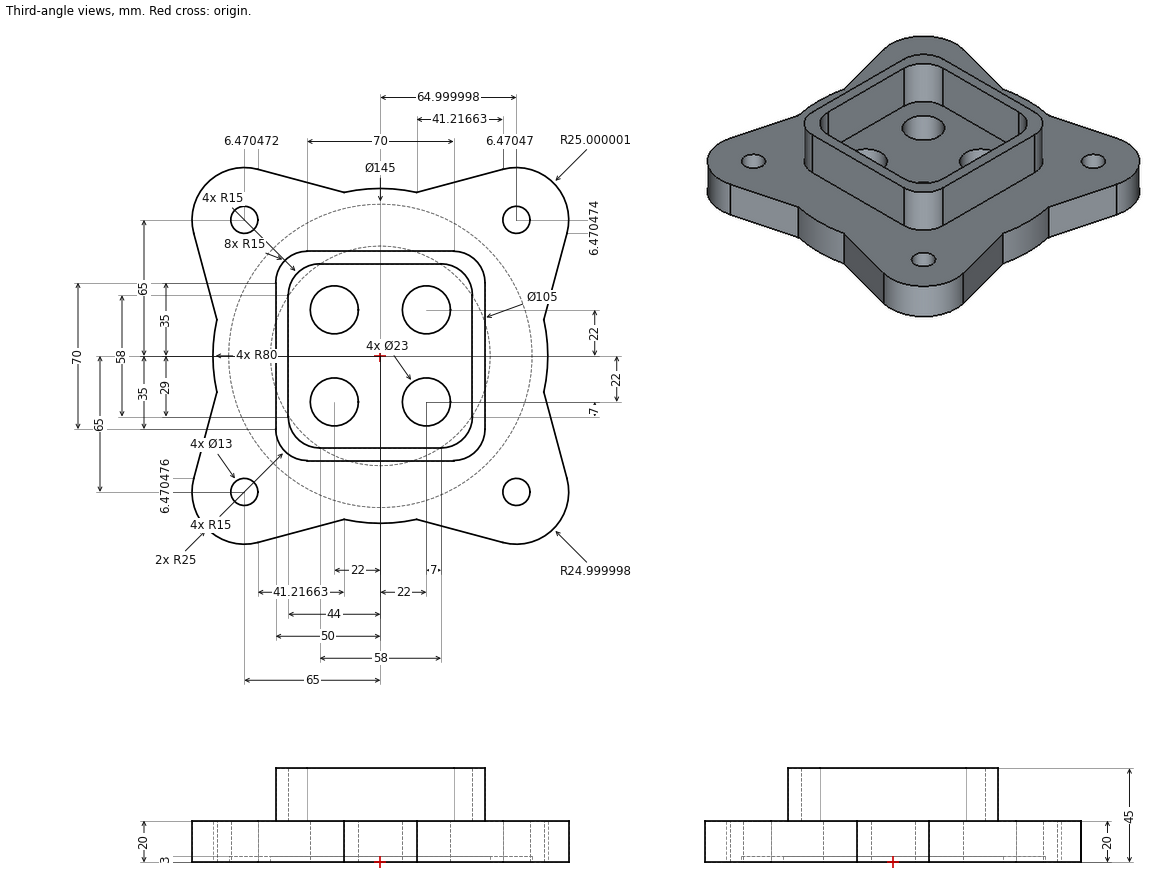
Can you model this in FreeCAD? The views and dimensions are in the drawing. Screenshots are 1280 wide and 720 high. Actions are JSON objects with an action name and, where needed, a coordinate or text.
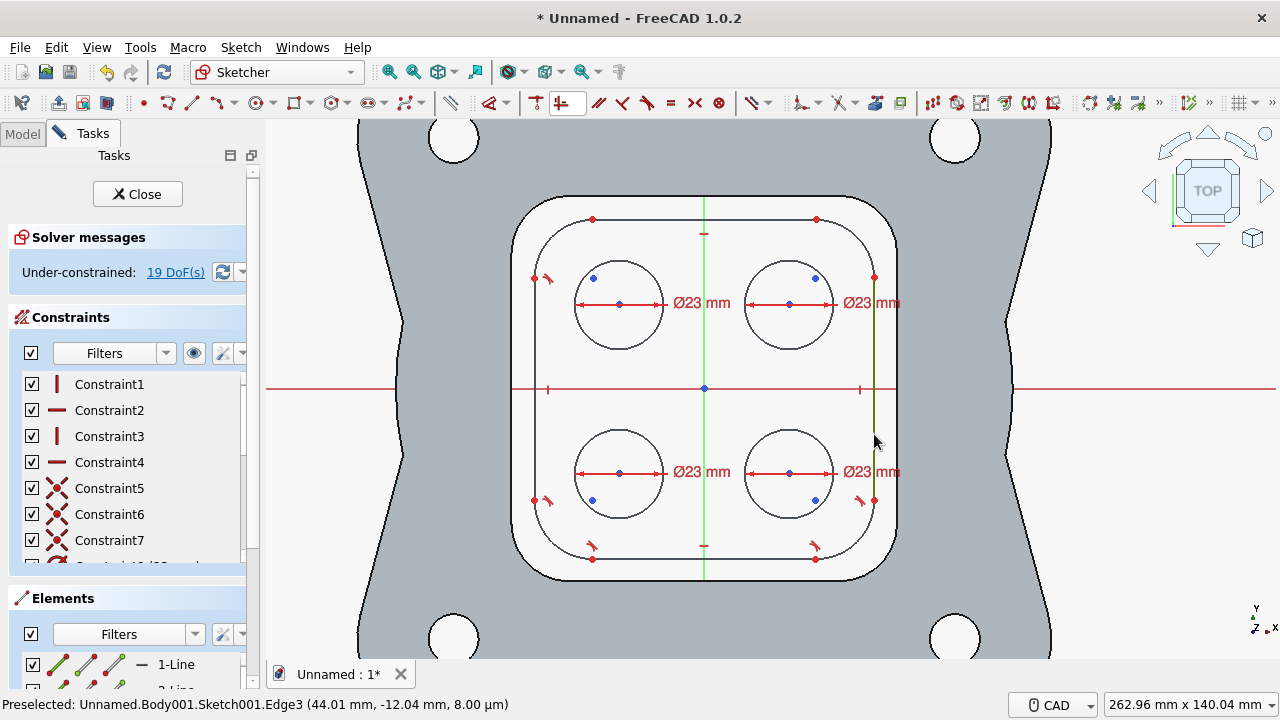
{"action": "left_click", "coordinate": [868, 252]}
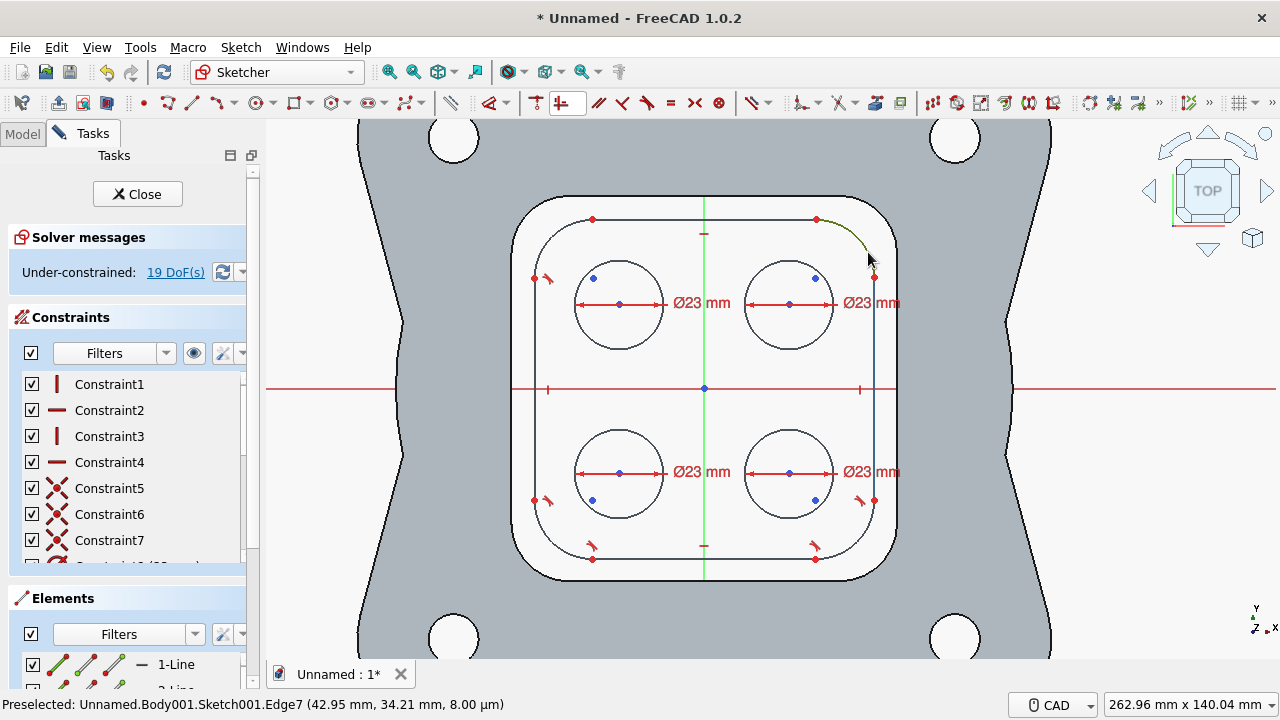
{"action": "key", "text": "t"}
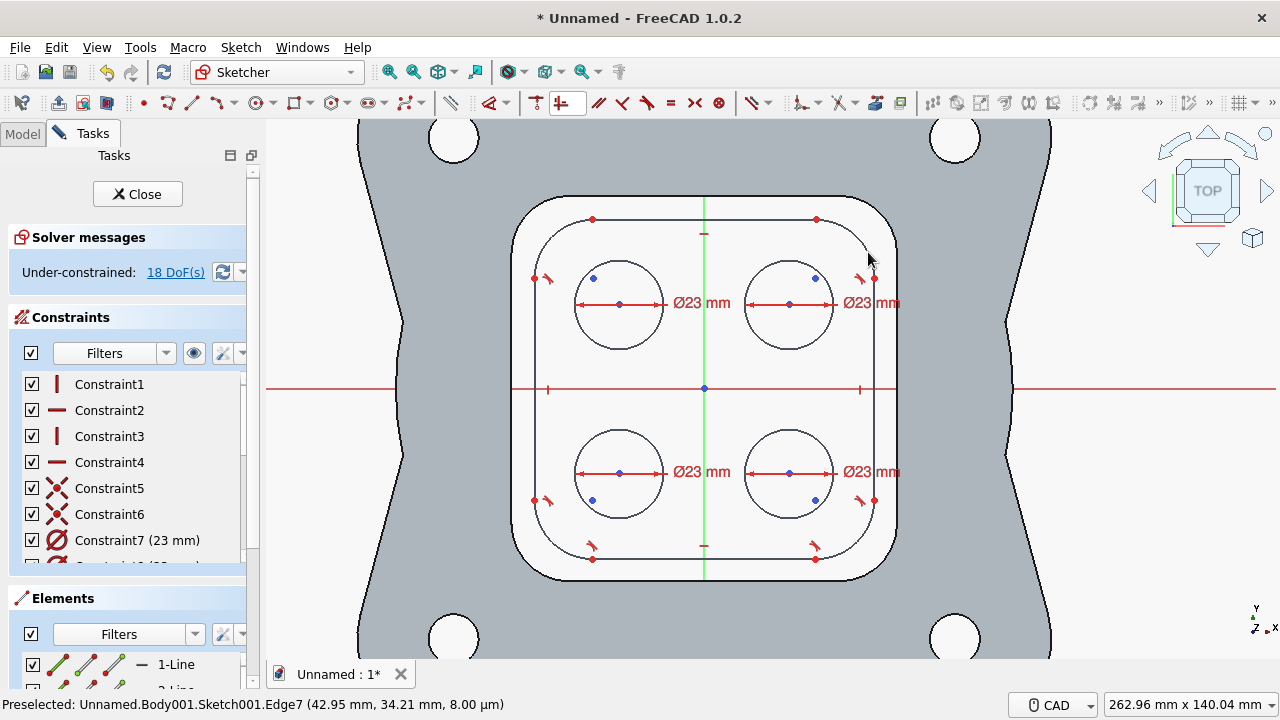
{"action": "left_click", "coordinate": [749, 220]}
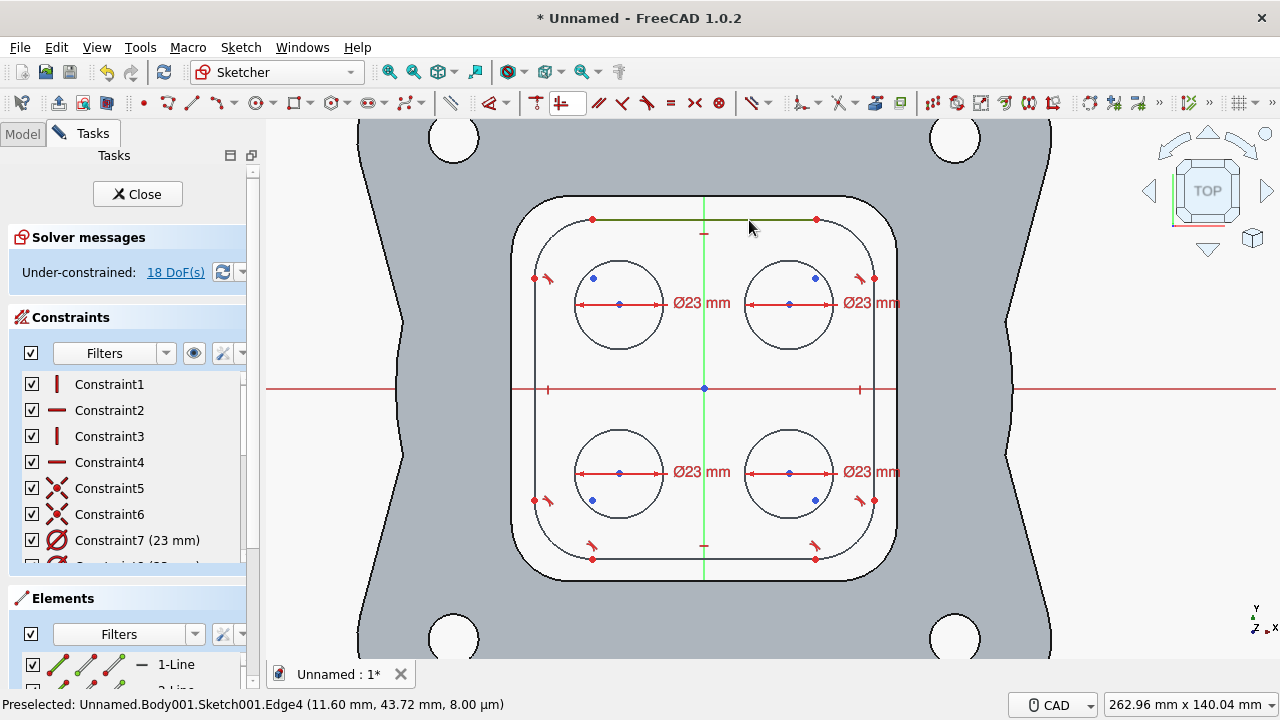
{"action": "left_click", "coordinate": [868, 252]}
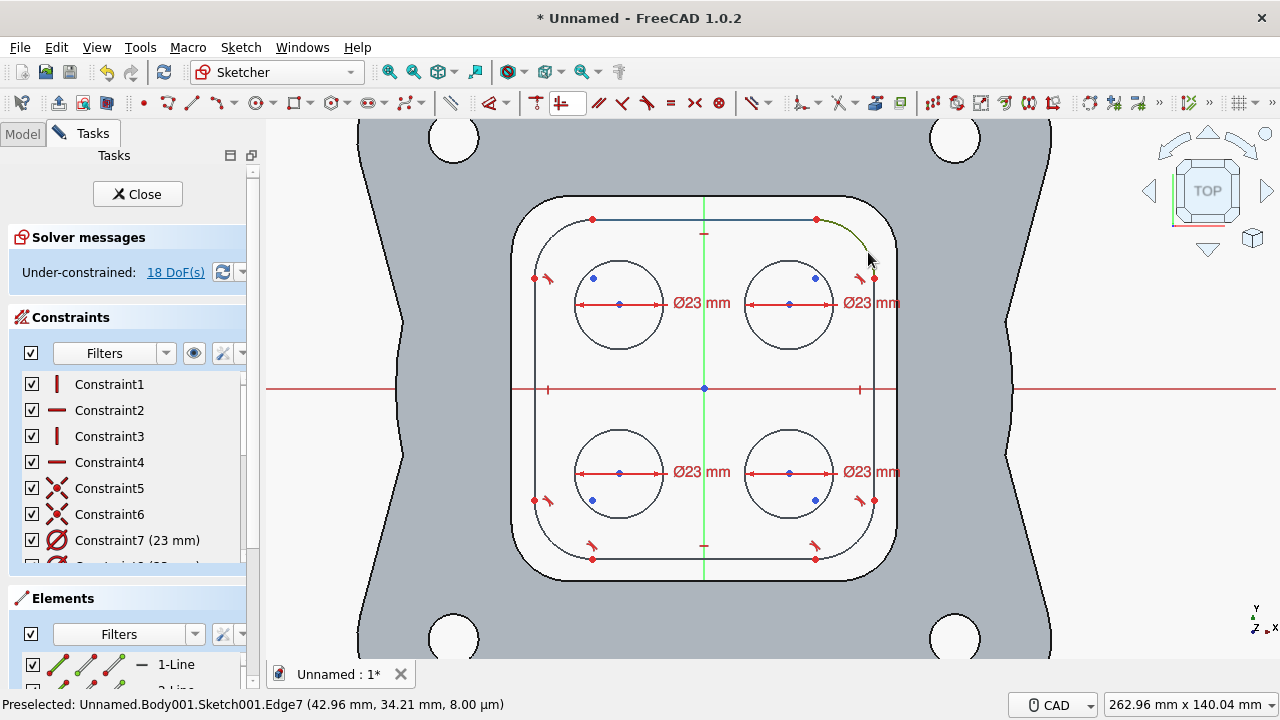
{"action": "left_click", "coordinate": [648, 104]}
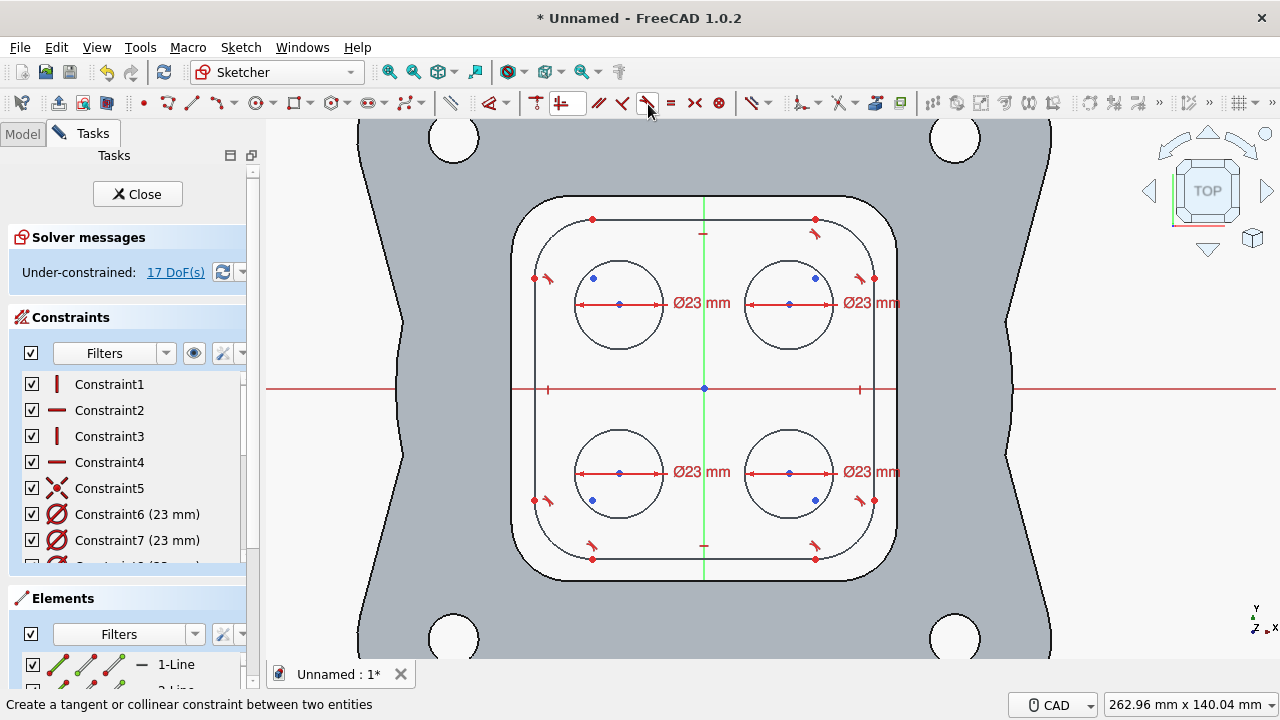
{"action": "left_click", "coordinate": [749, 220]}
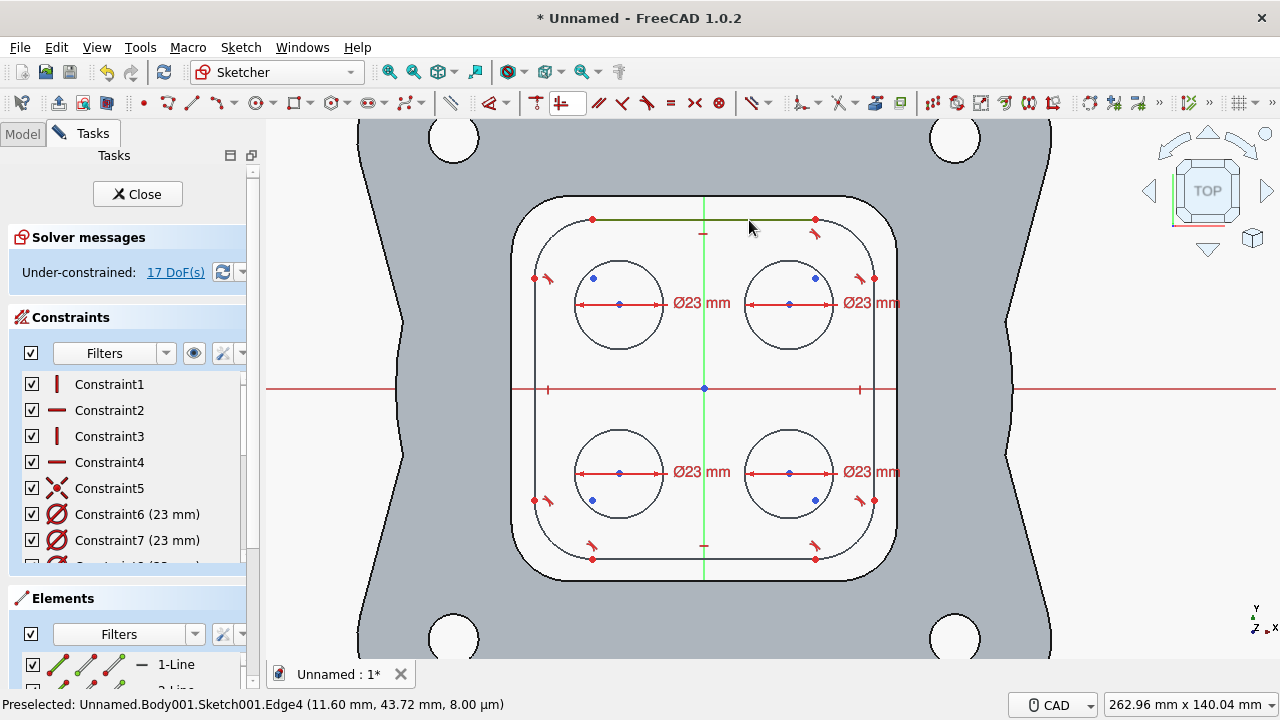
{"action": "left_click", "coordinate": [566, 227]}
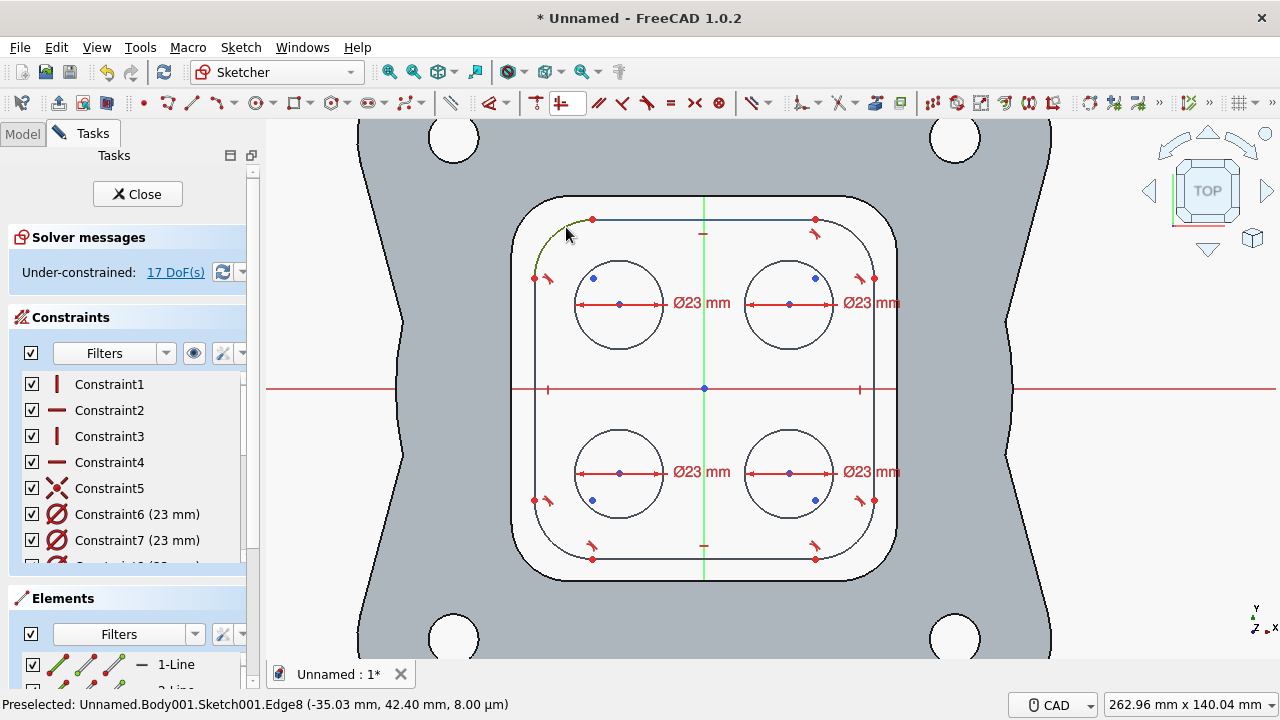
{"action": "left_click", "coordinate": [648, 104]}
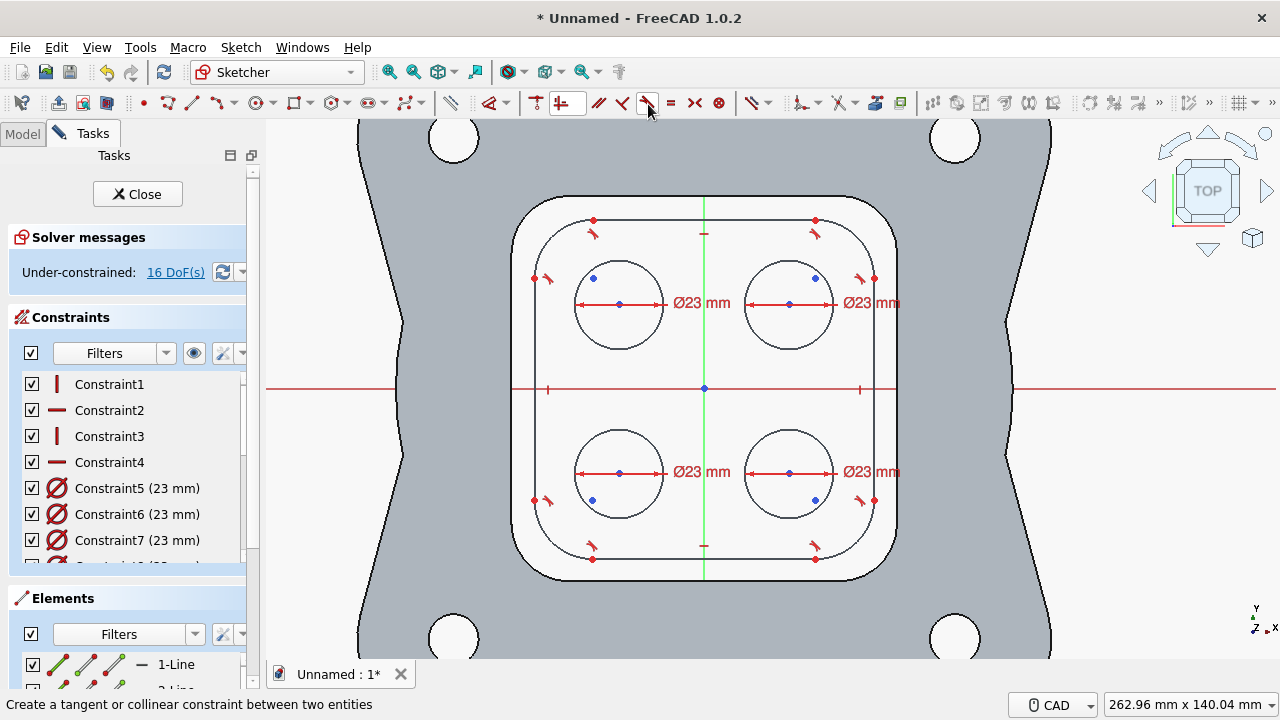
{"action": "left_click", "coordinate": [541, 527]}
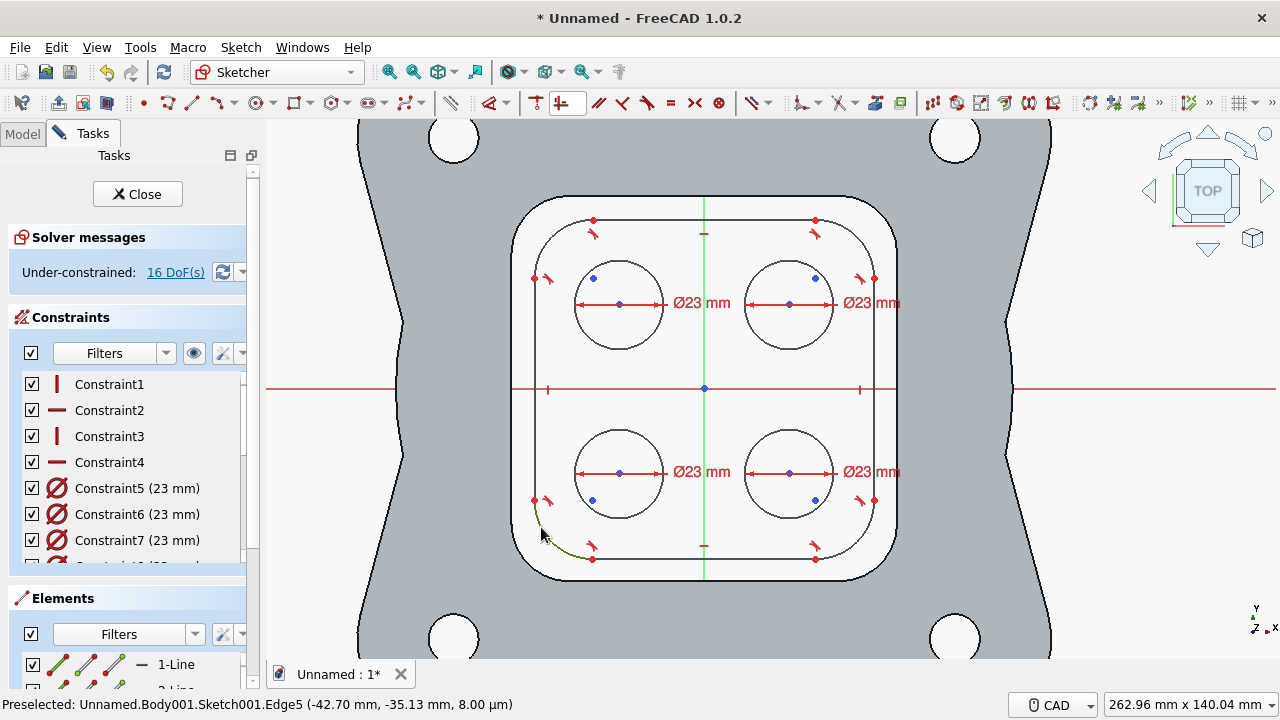
{"action": "left_click", "coordinate": [842, 553]}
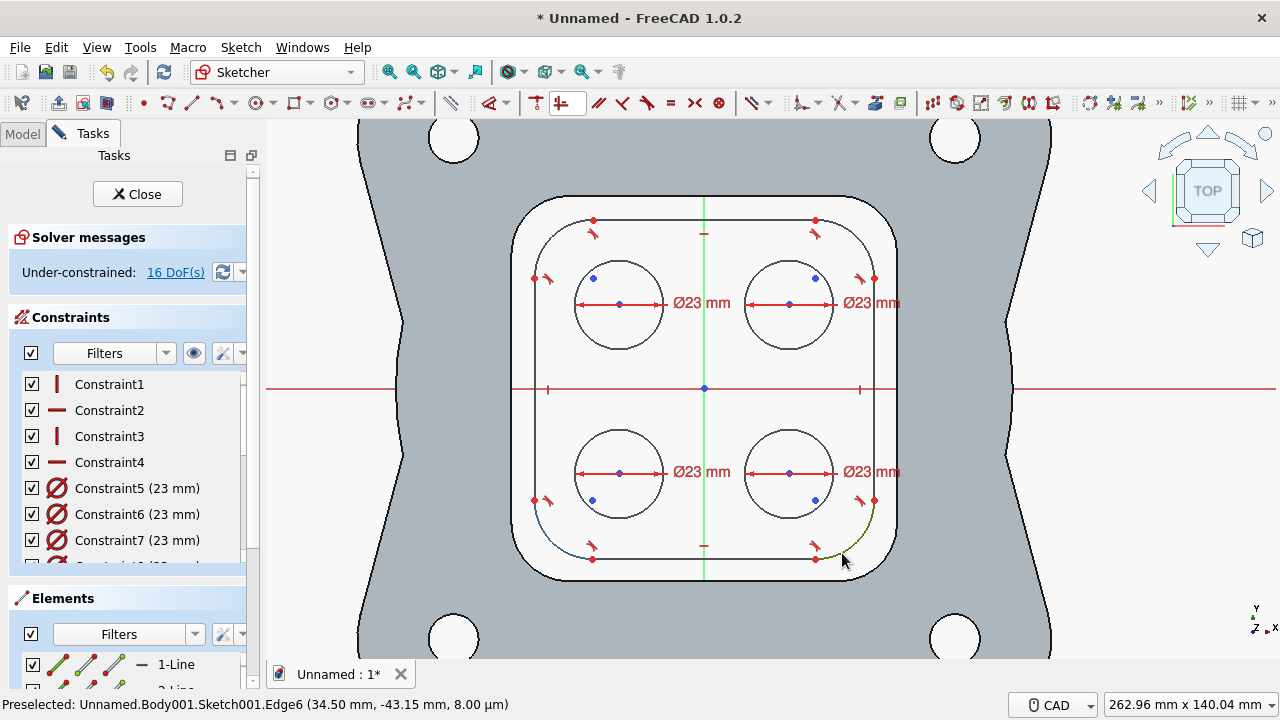
{"action": "left_click", "coordinate": [868, 252]}